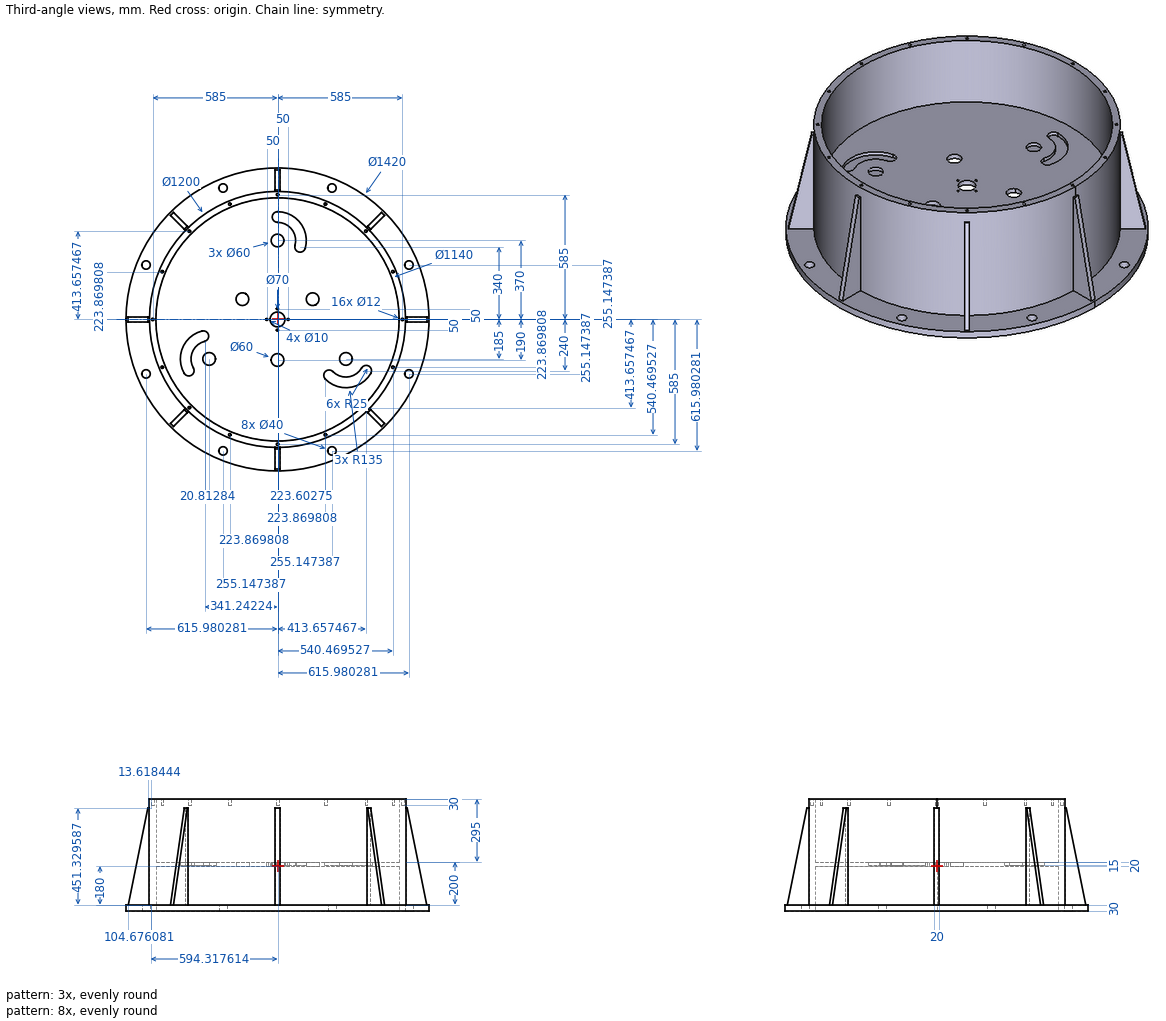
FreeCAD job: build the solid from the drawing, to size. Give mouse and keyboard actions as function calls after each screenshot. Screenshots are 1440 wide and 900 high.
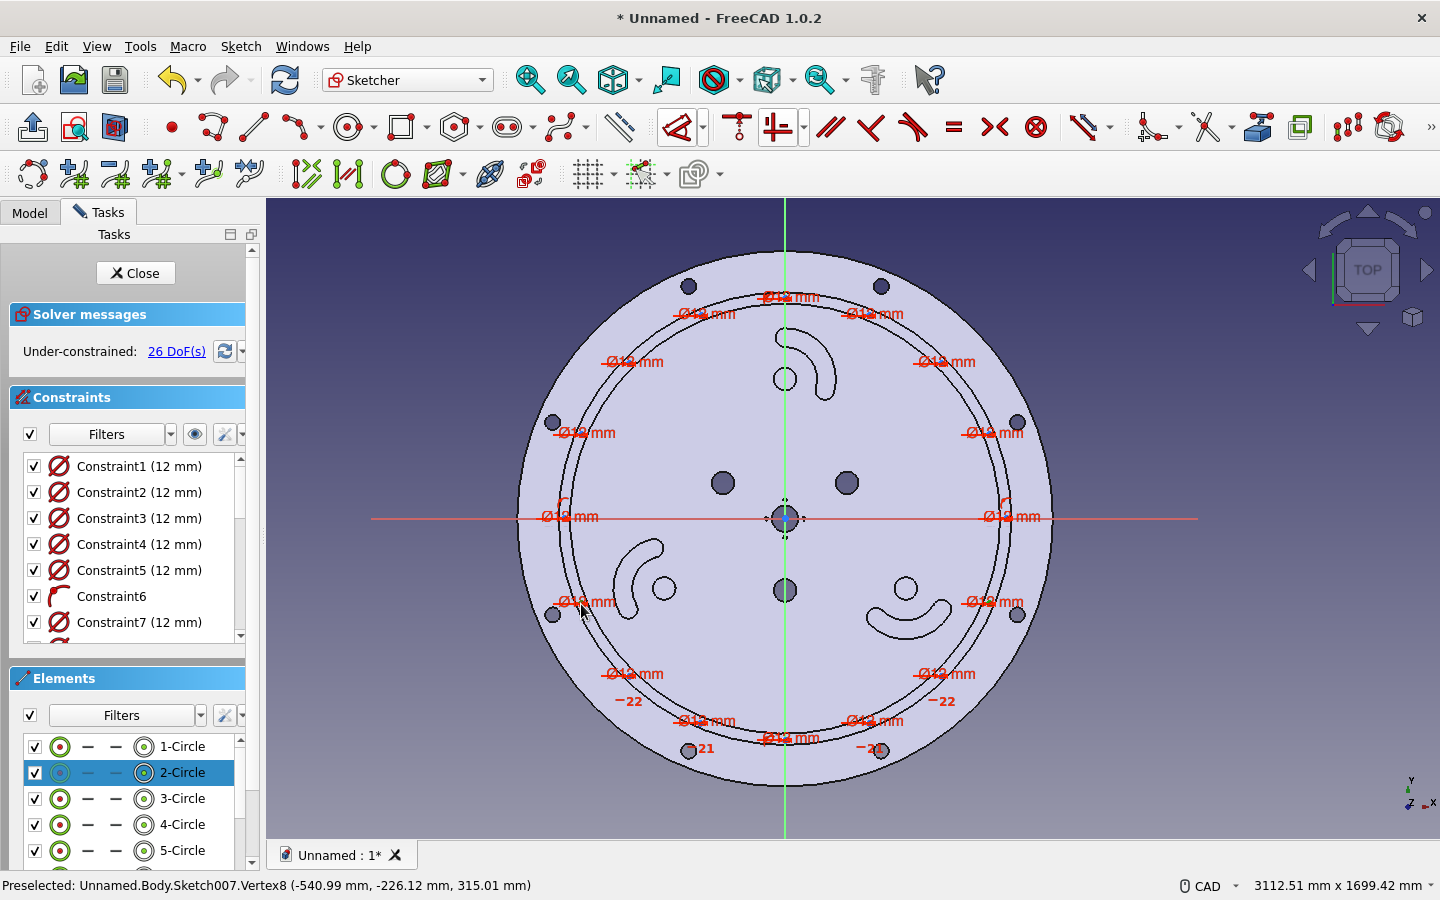
key(h)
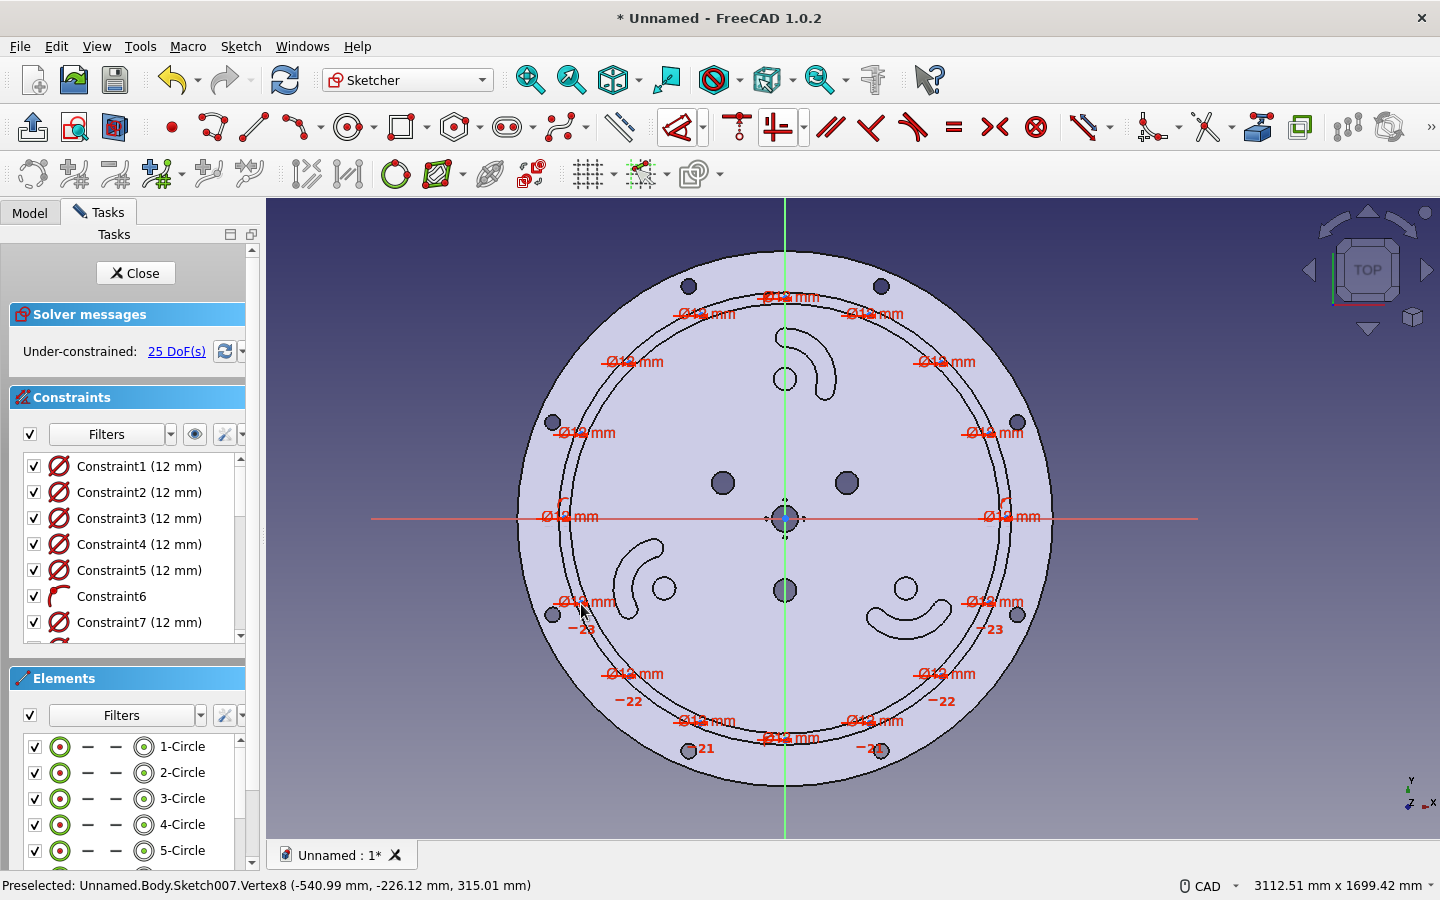
click(581, 604)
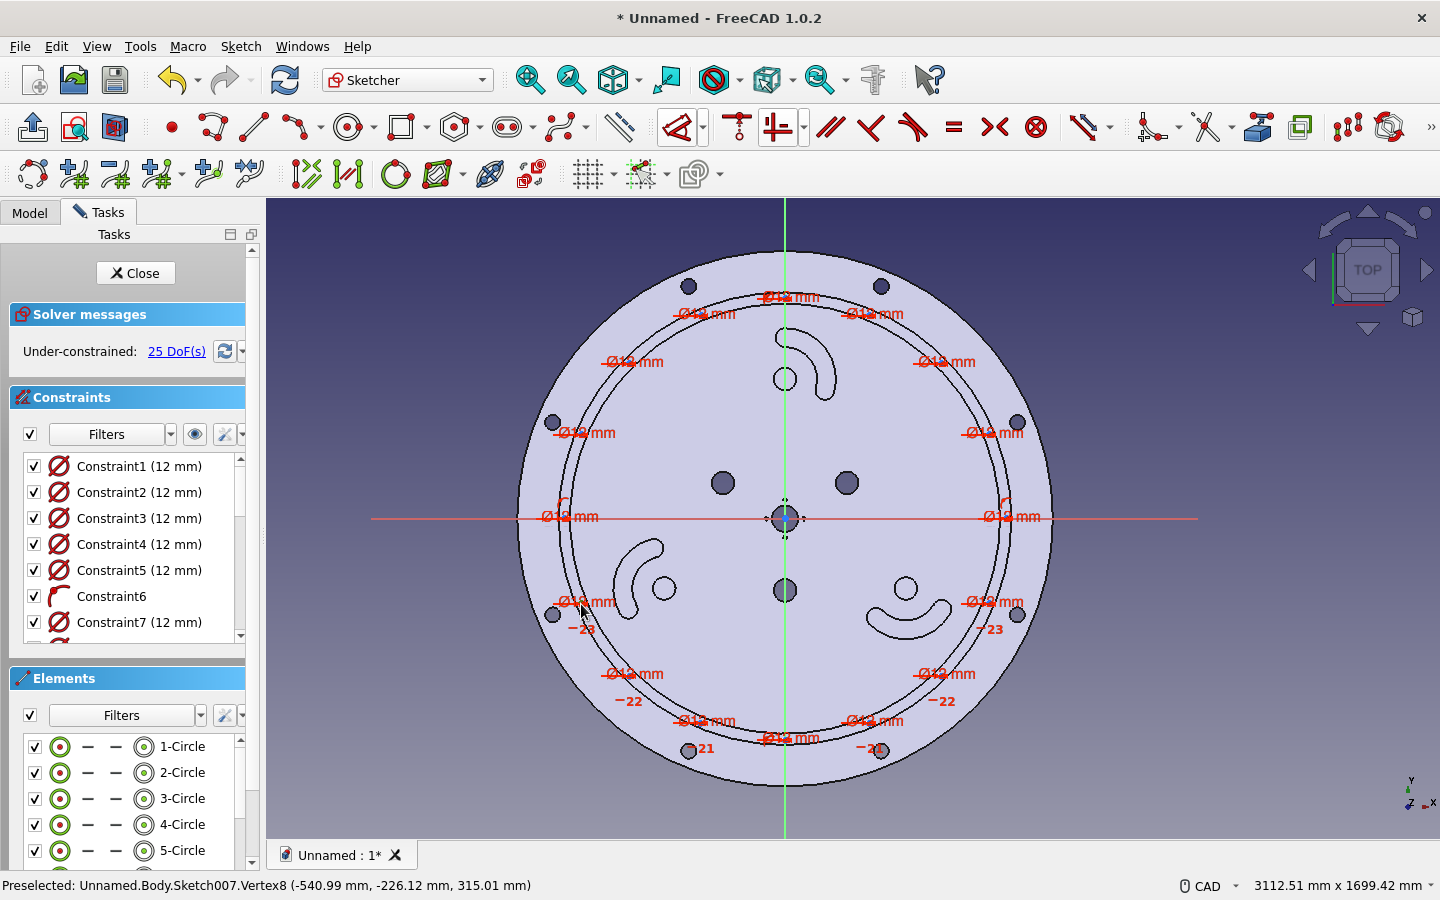
click(581, 435)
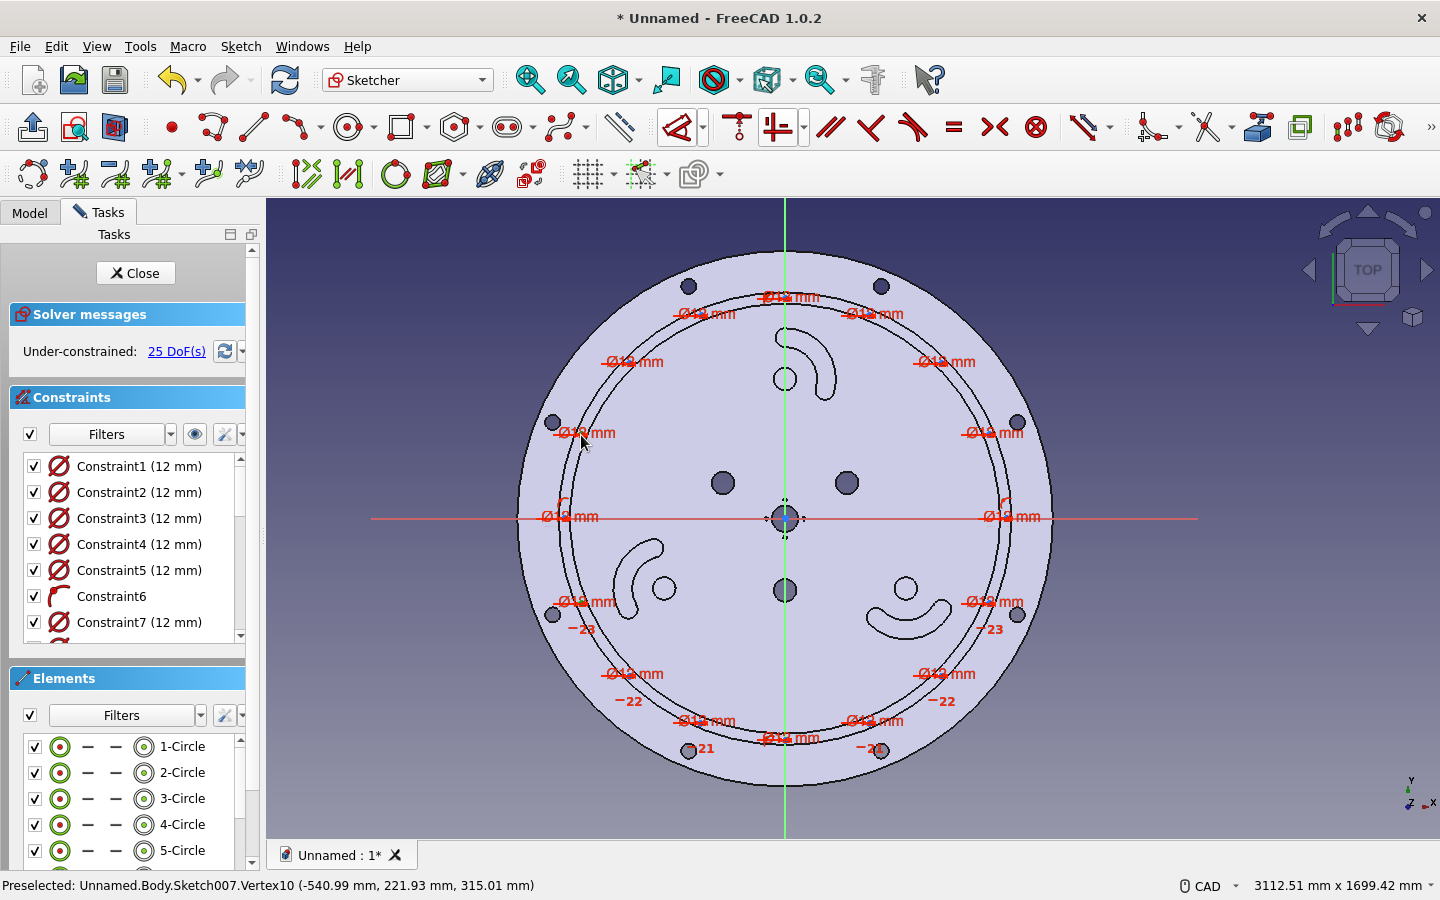
key(v)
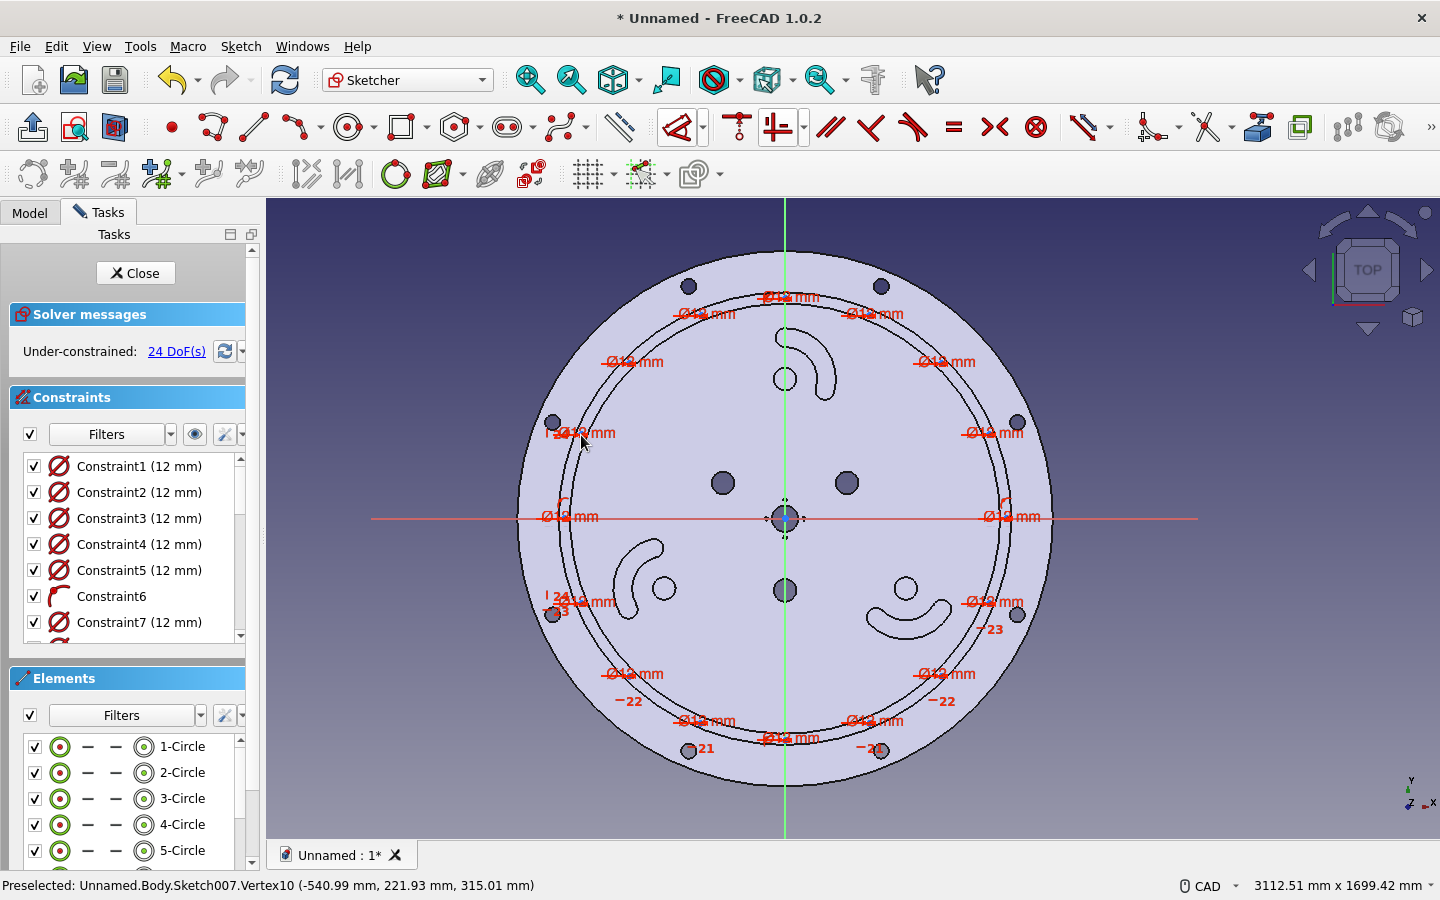
click(629, 676)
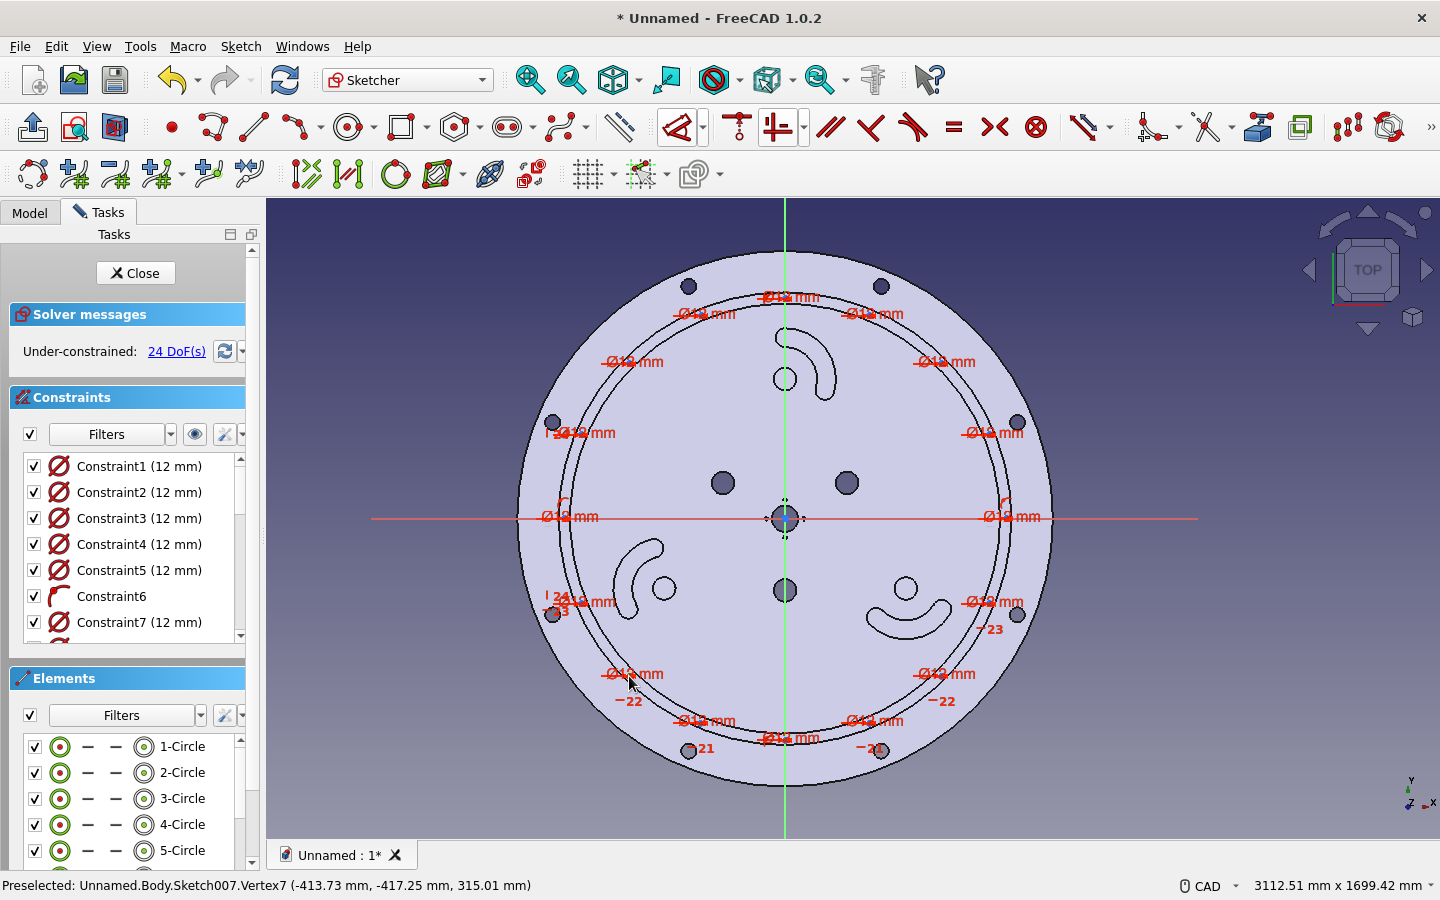
click(629, 364)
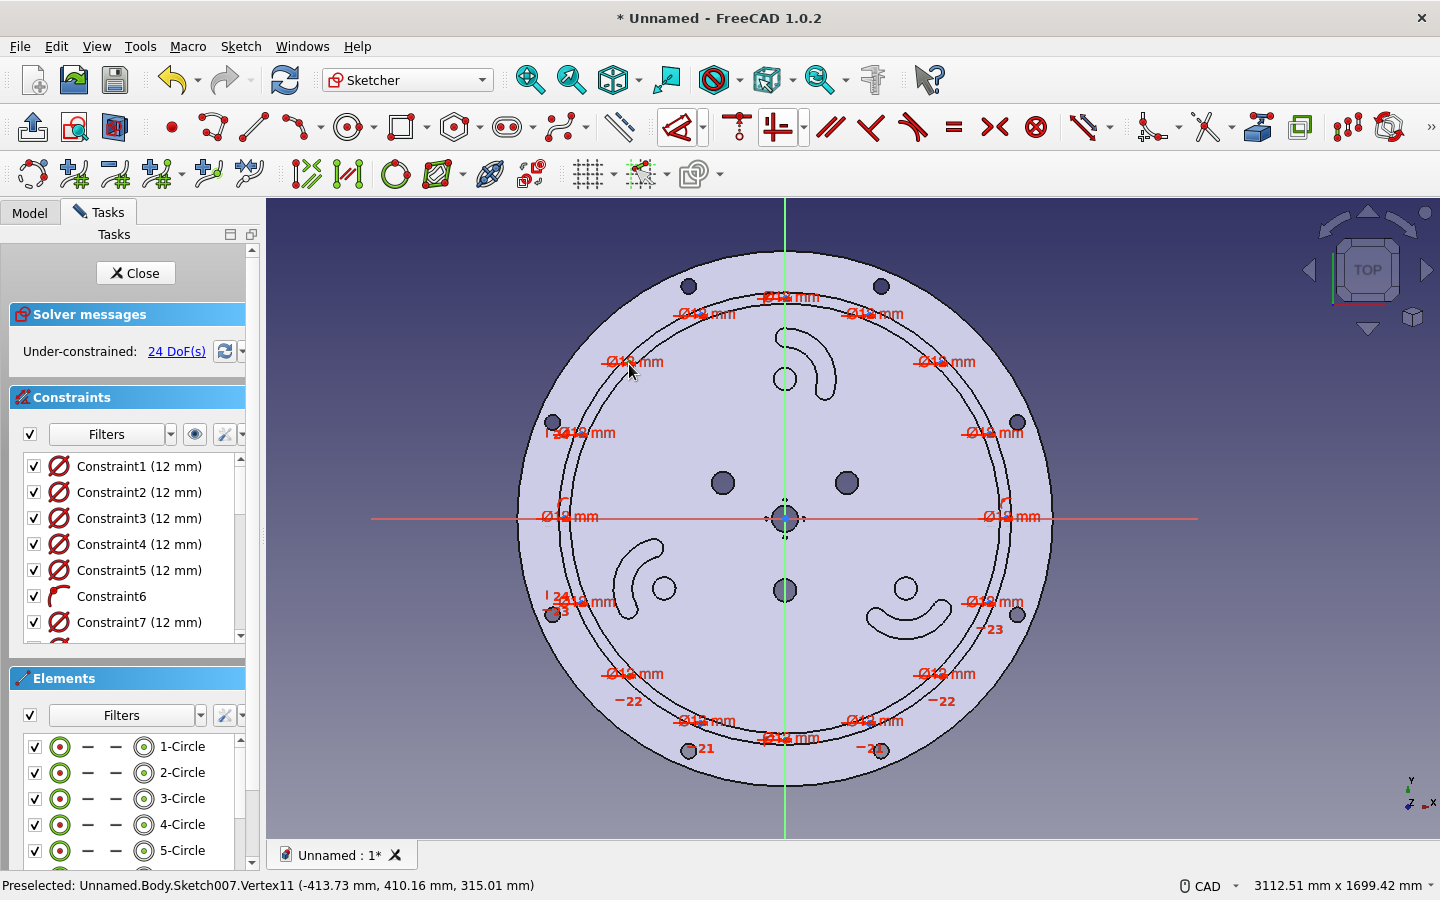
key(v)